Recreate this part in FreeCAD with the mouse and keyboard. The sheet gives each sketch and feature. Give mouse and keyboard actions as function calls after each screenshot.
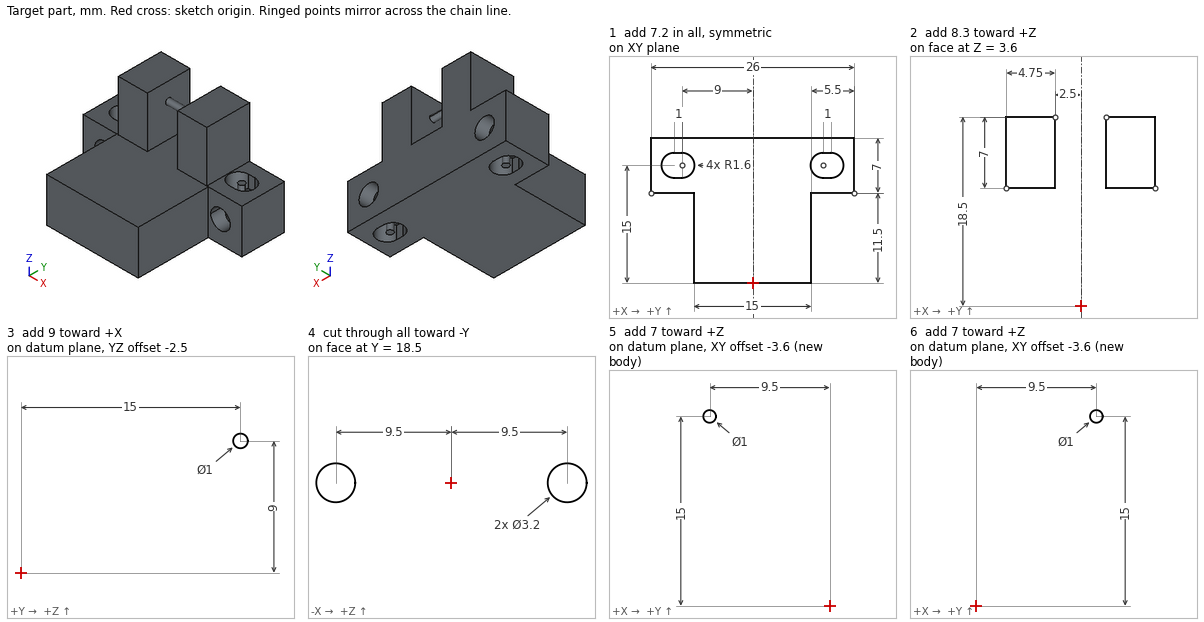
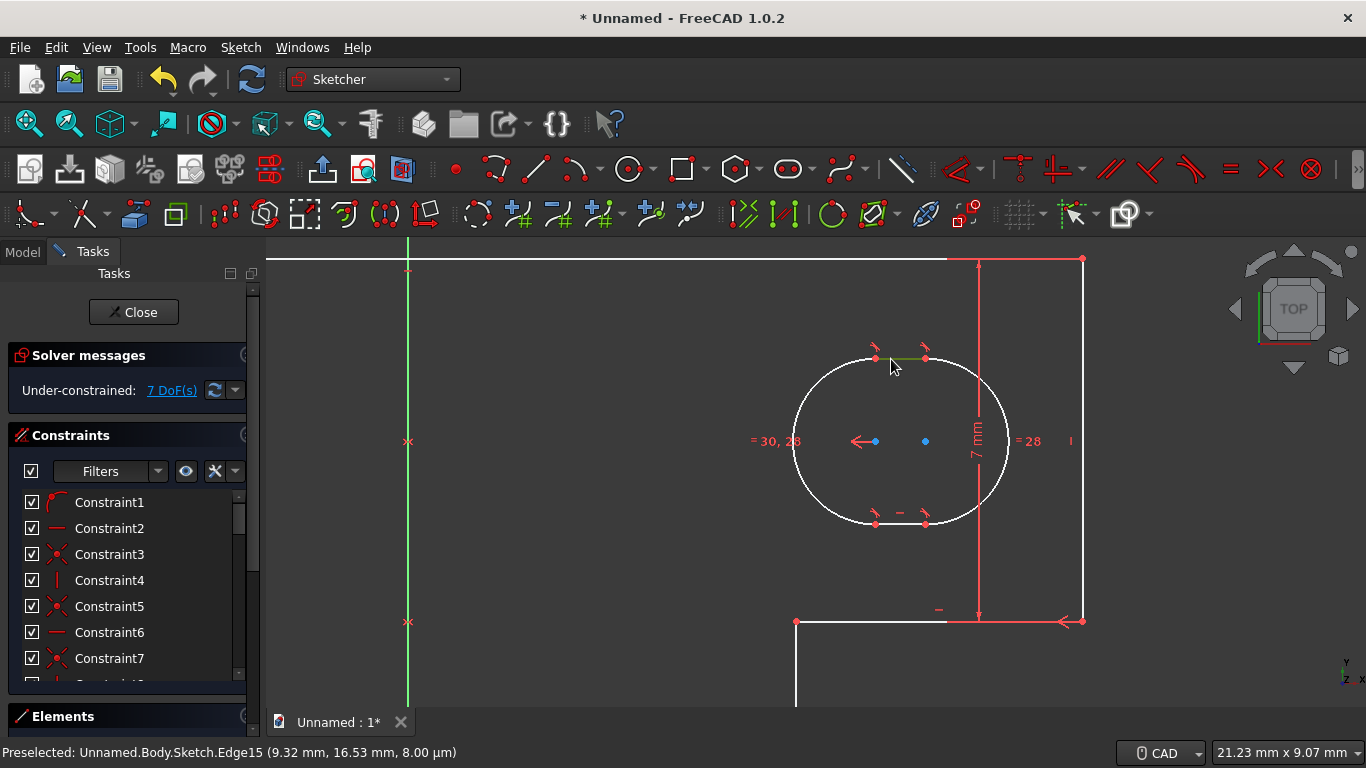
click(982, 170)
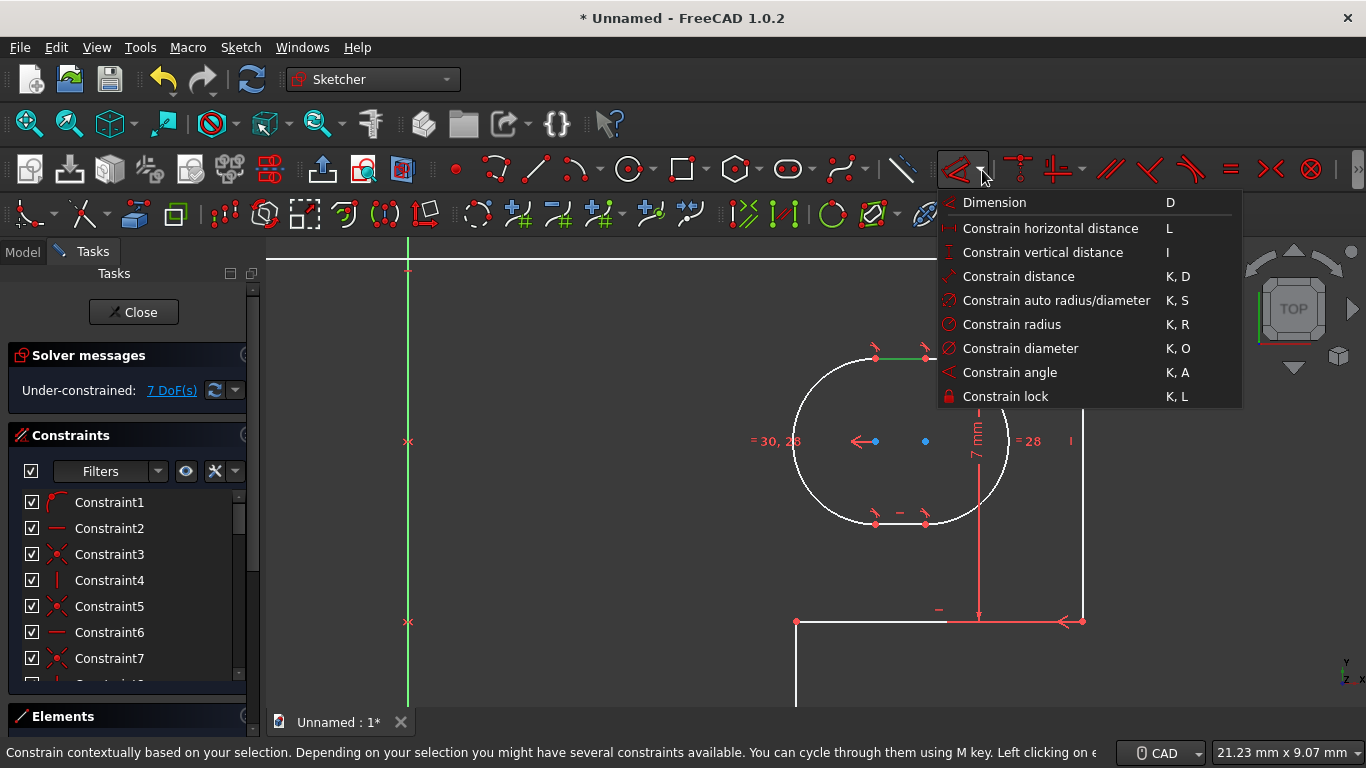
click(1090, 228)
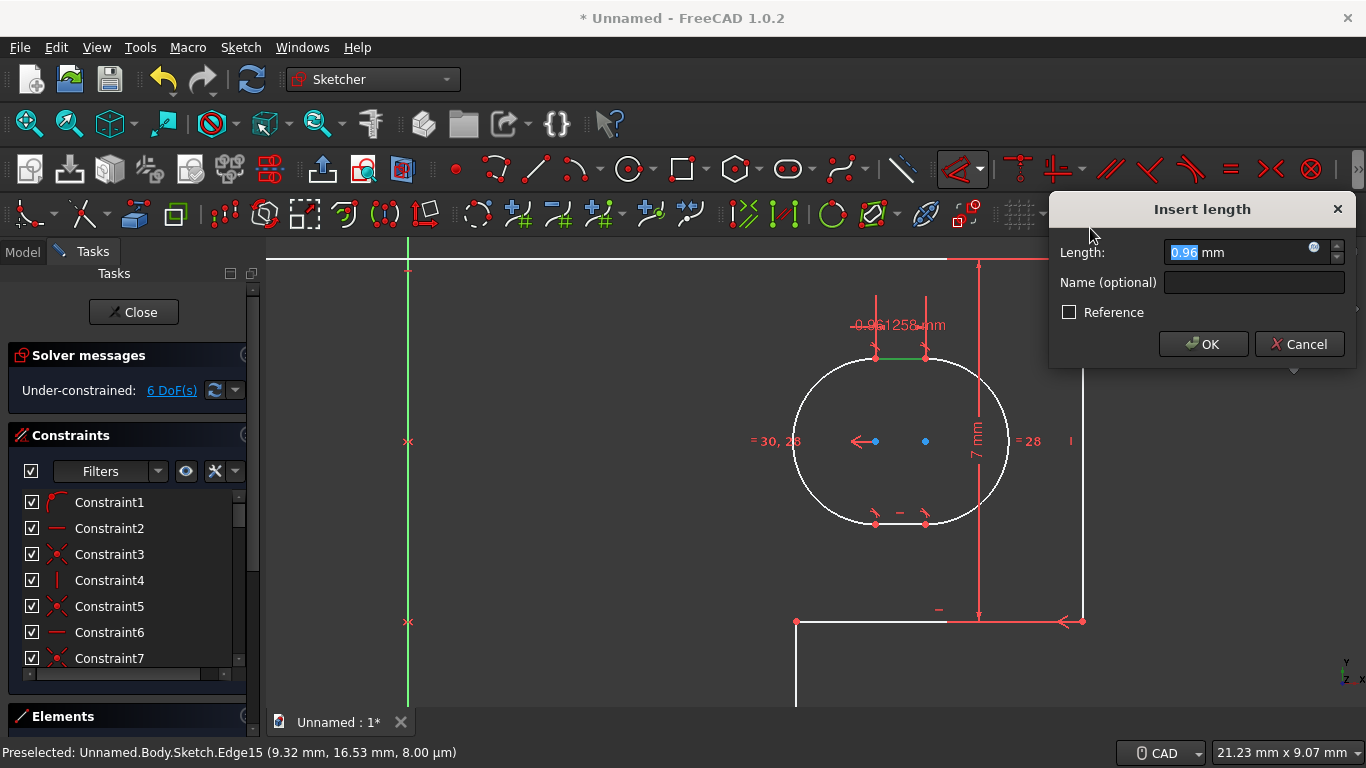
text(1)
key(Return)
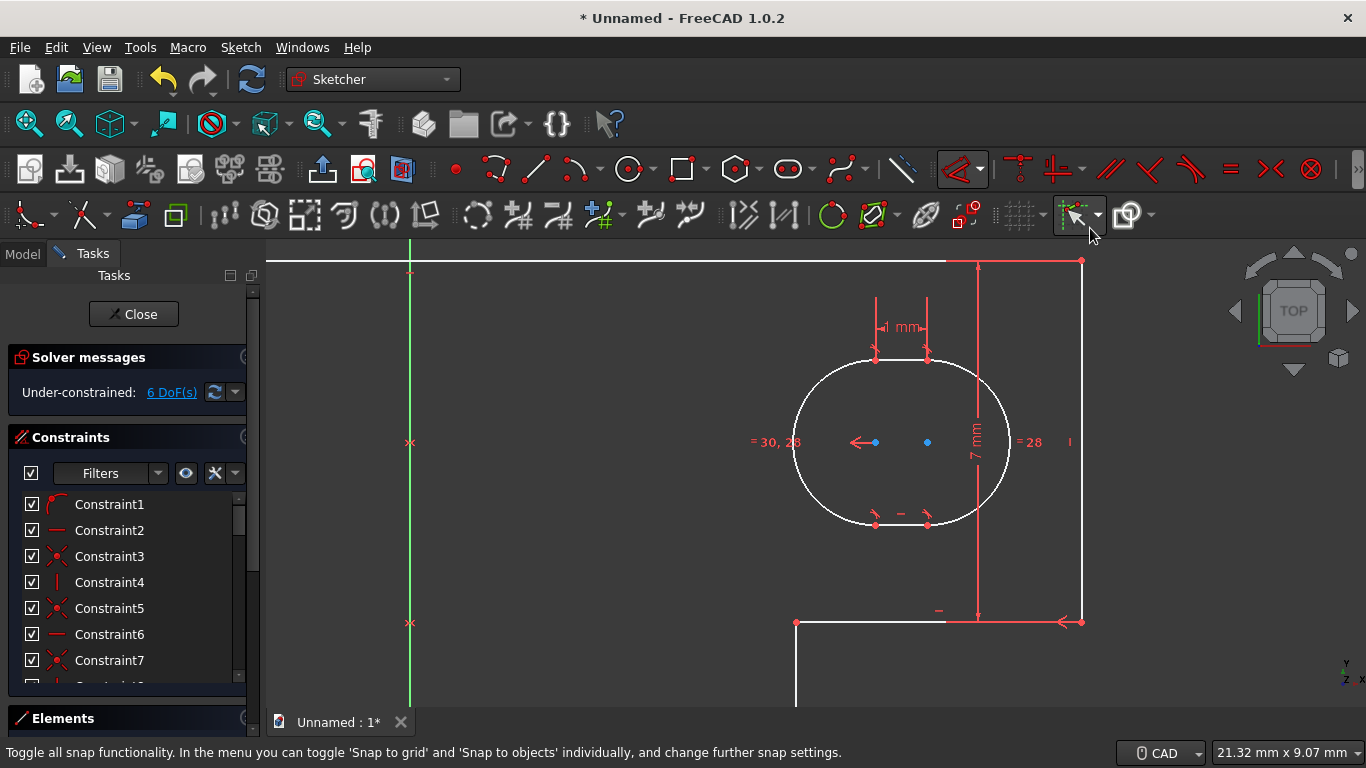
scroll(893, 360, down, 6)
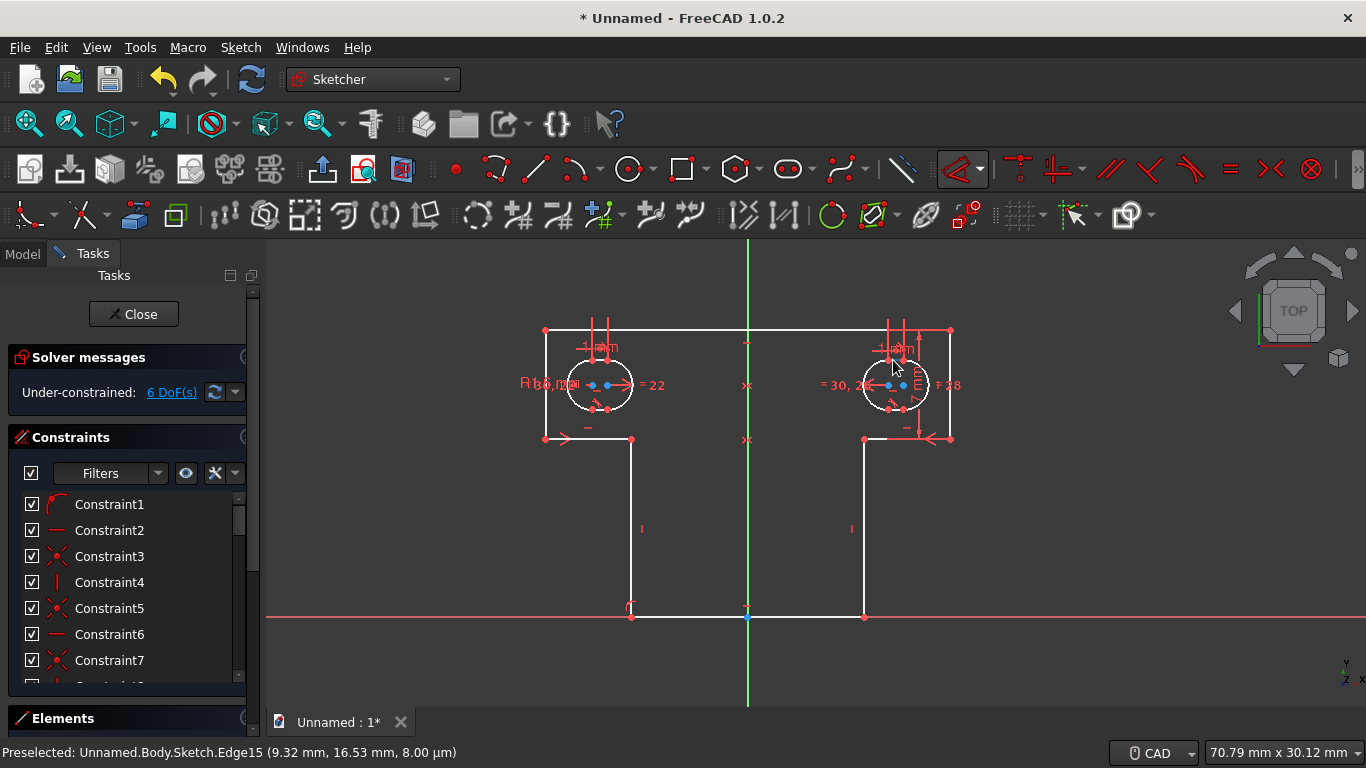
click(701, 617)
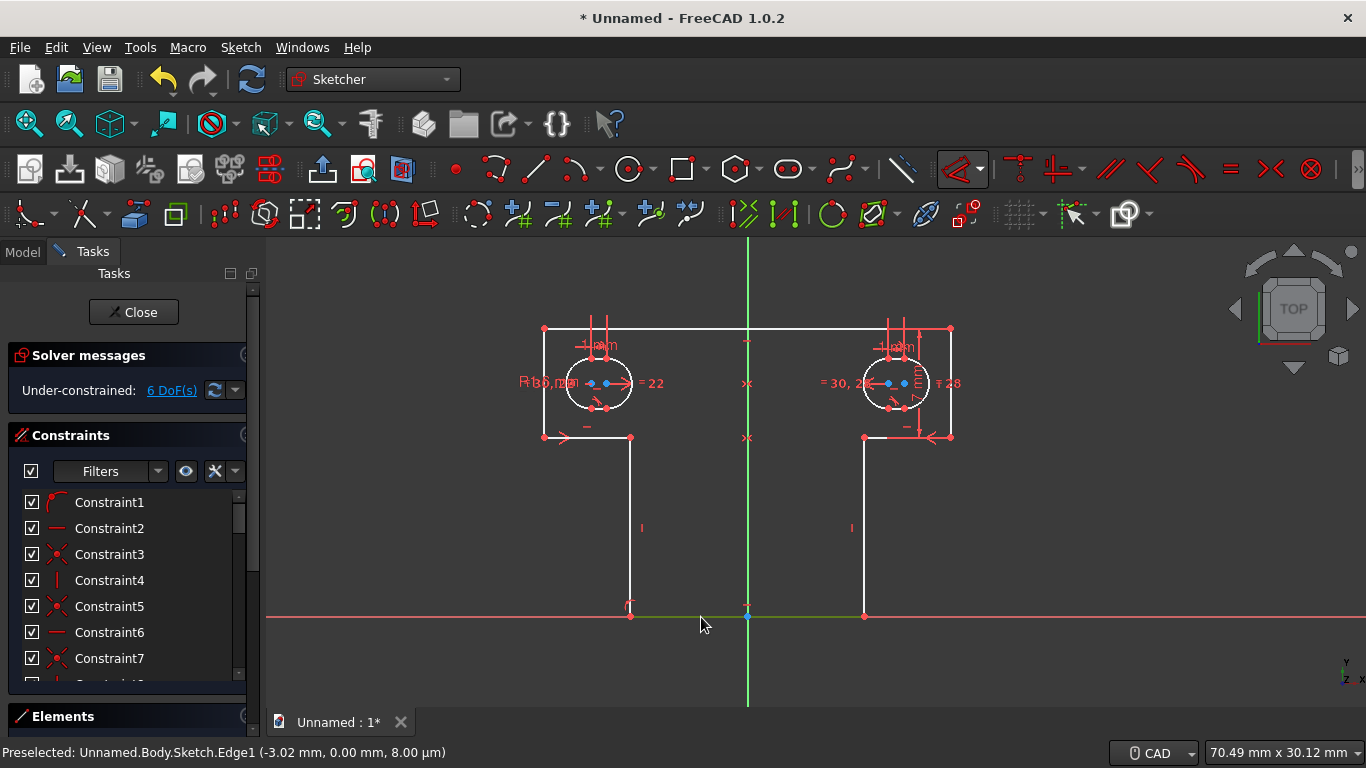
key(l)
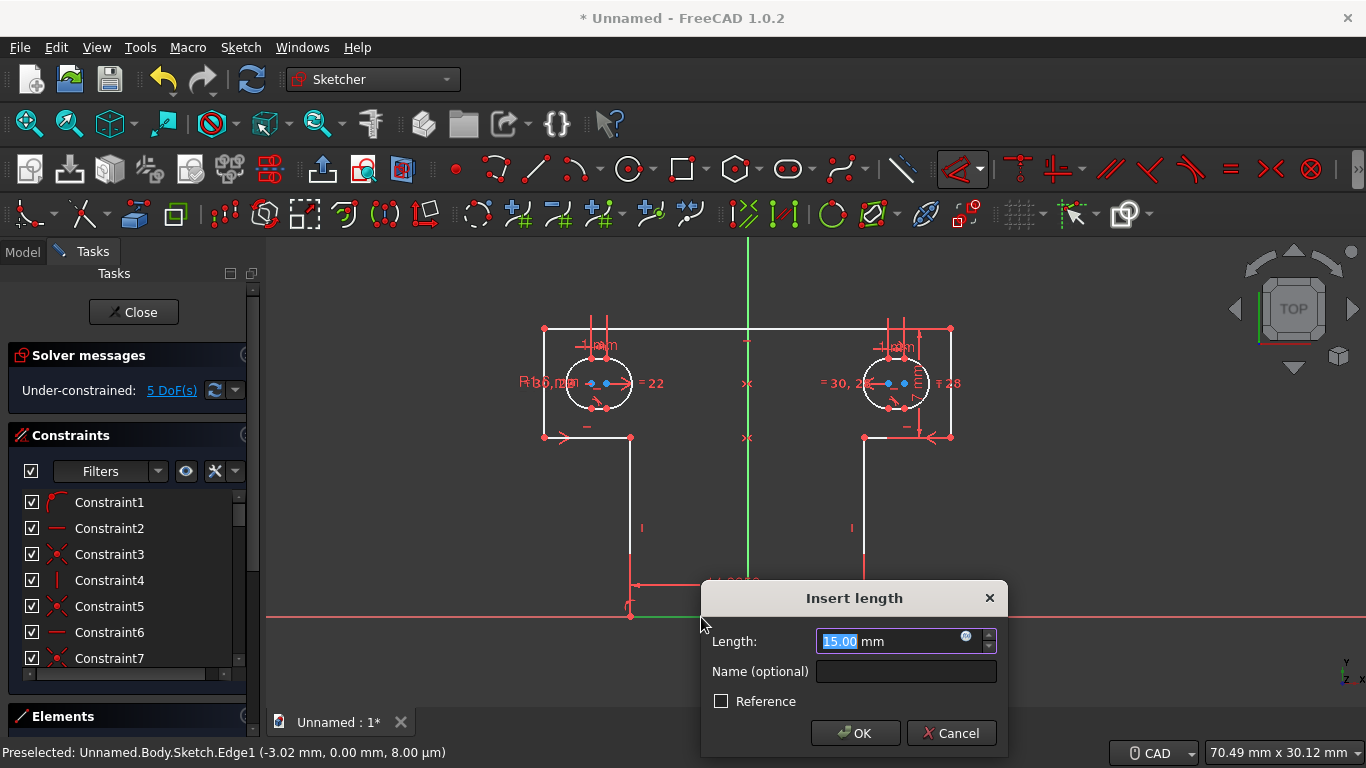
text(15)
key(Return)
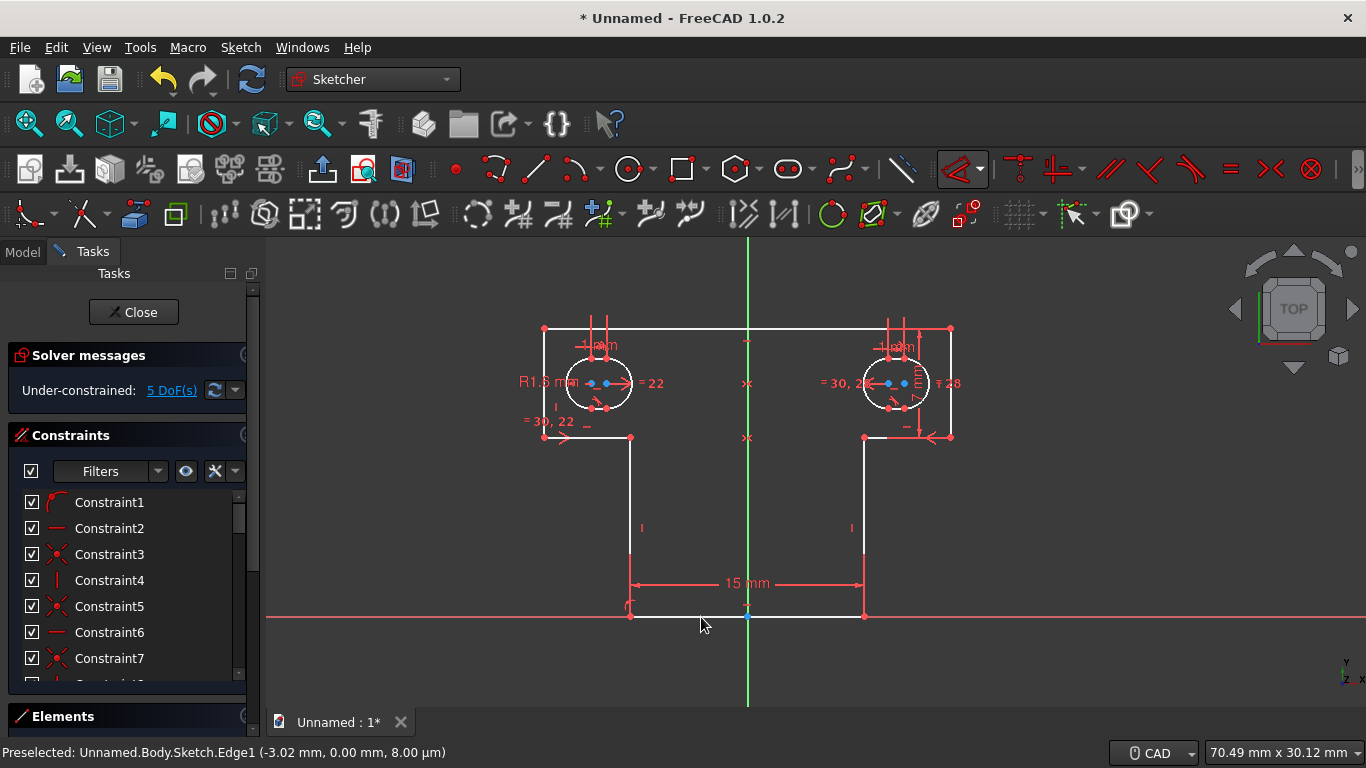
click(829, 329)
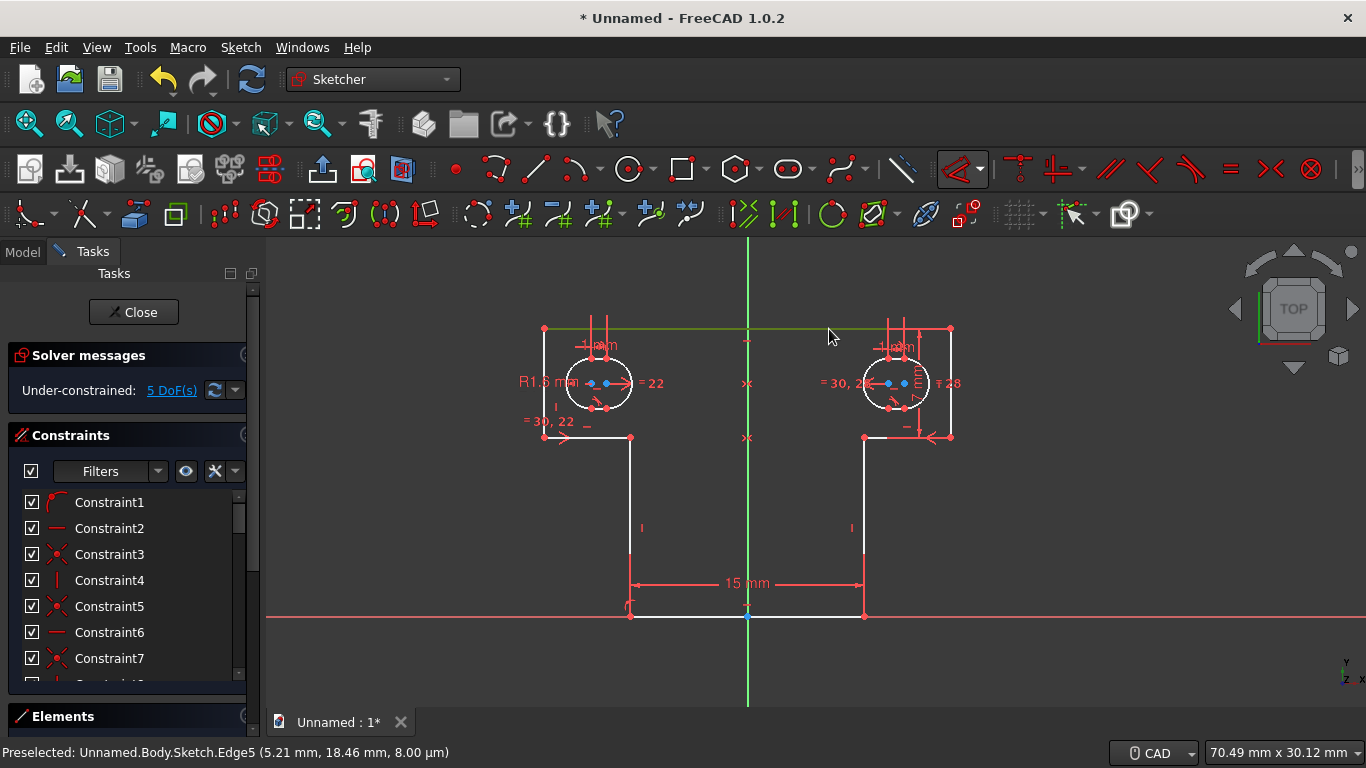
key(l)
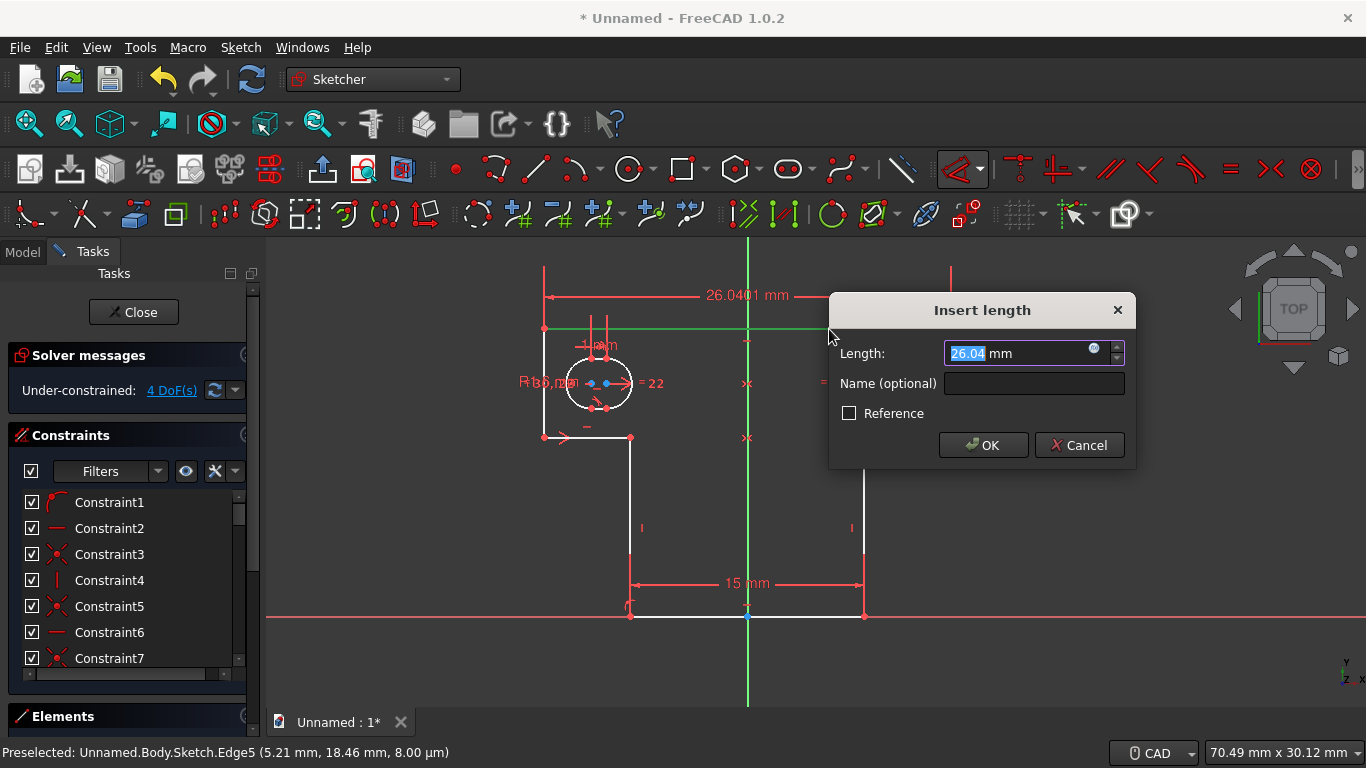
text(26)
key(Return)